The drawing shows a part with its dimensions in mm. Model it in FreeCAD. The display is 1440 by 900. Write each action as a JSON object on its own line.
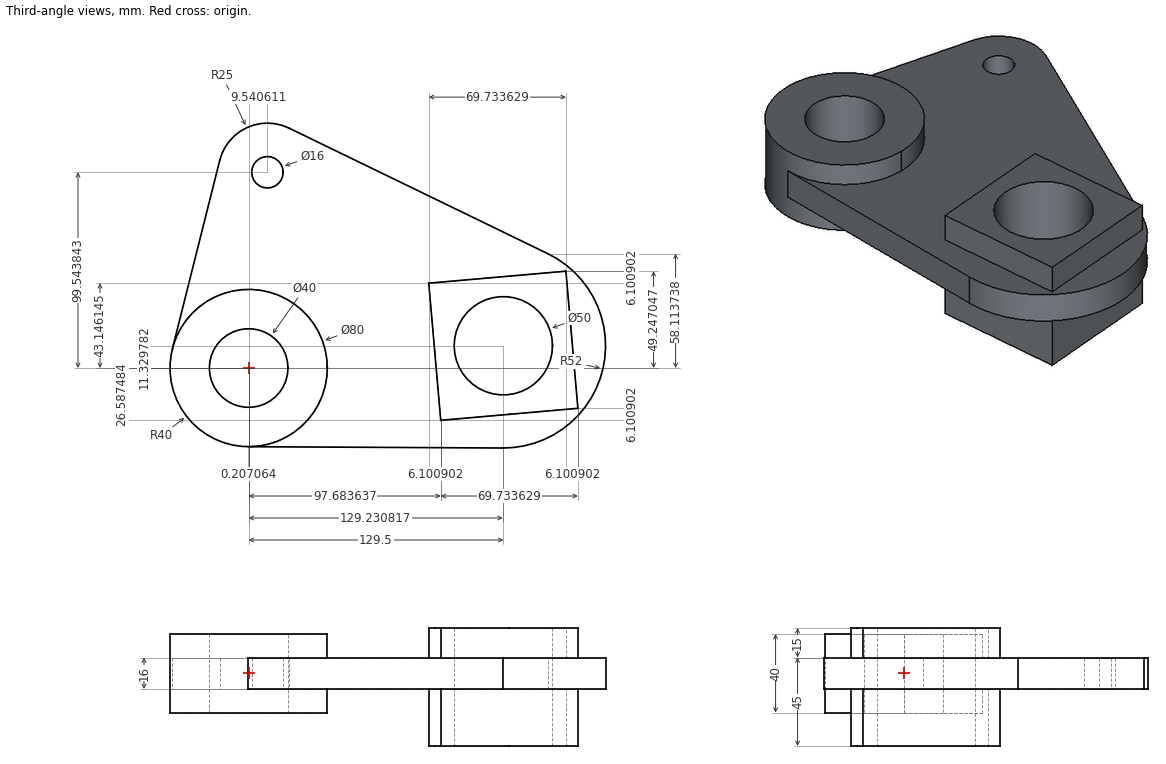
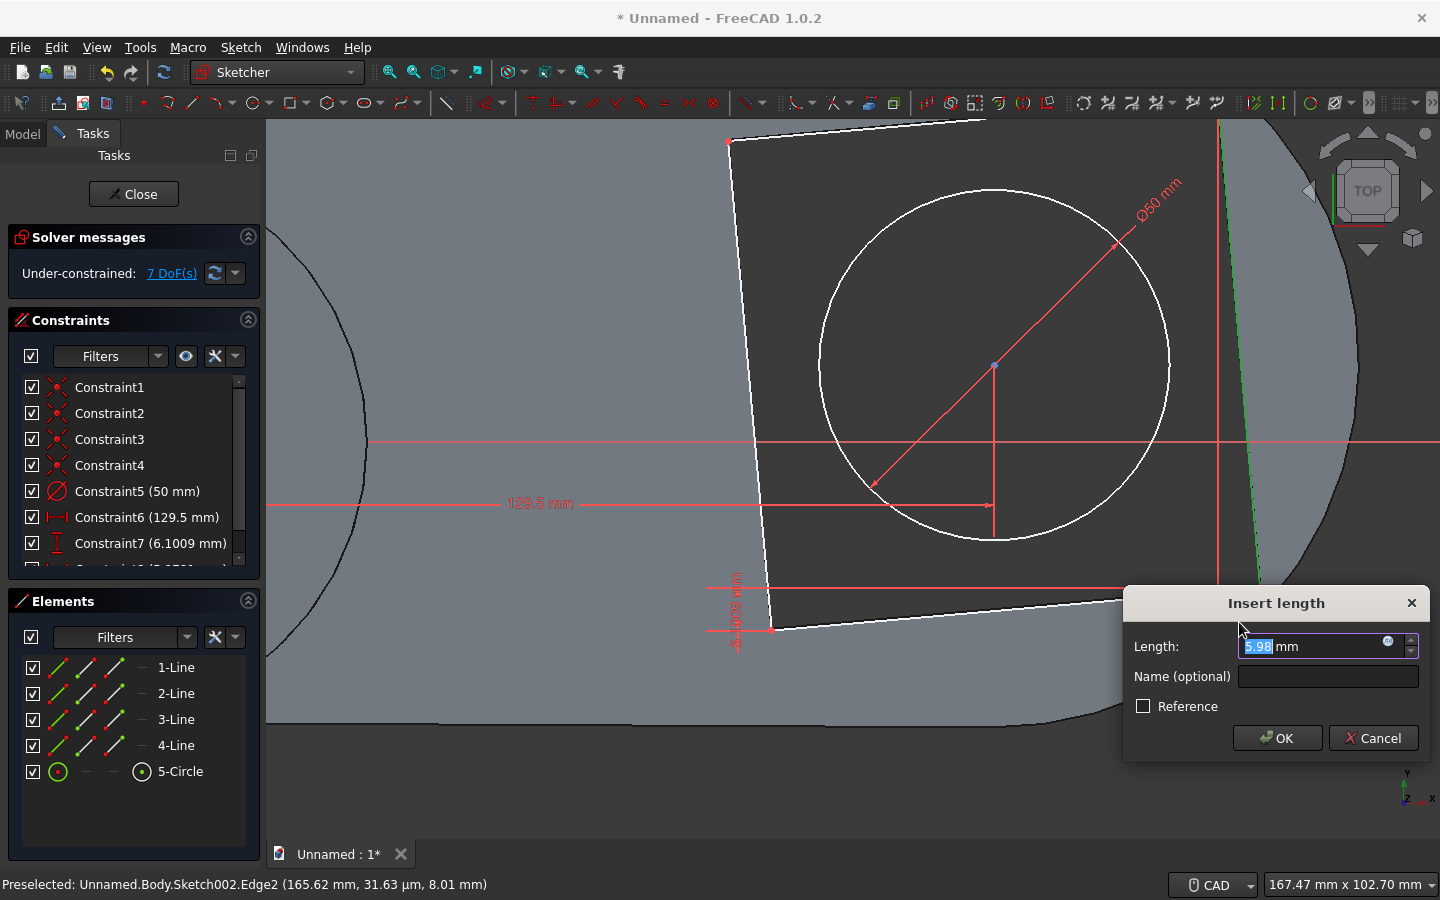
{"action": "type", "text": "6.100902"}
{"action": "key", "text": "Return"}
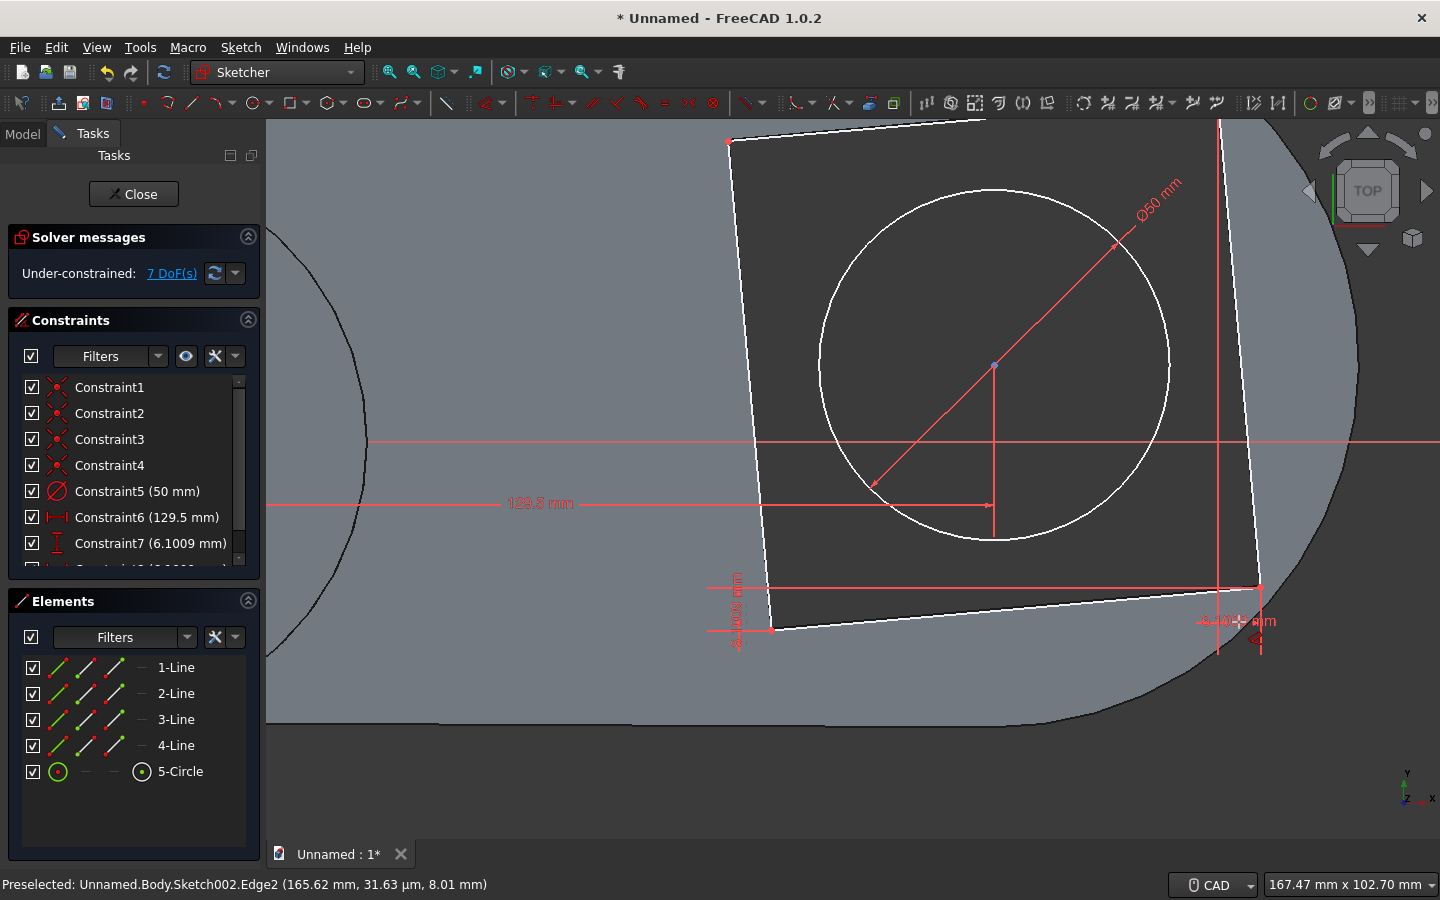
{"action": "scroll", "coordinate": [920, 620], "scroll_direction": "down", "scroll_amount": 3}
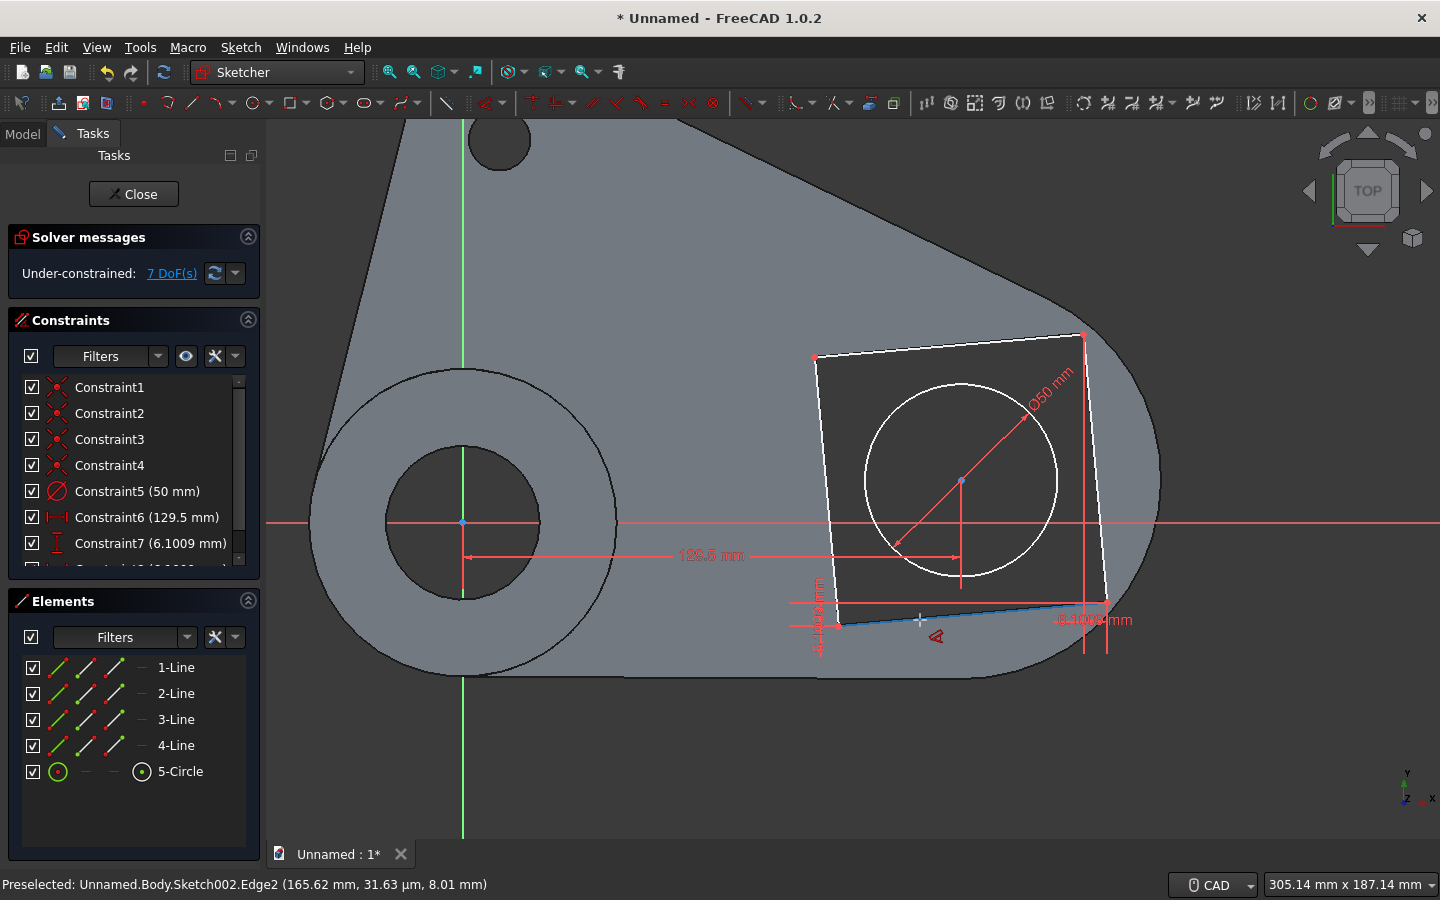
{"action": "scroll", "coordinate": [1003, 341], "scroll_direction": "up", "scroll_amount": 3}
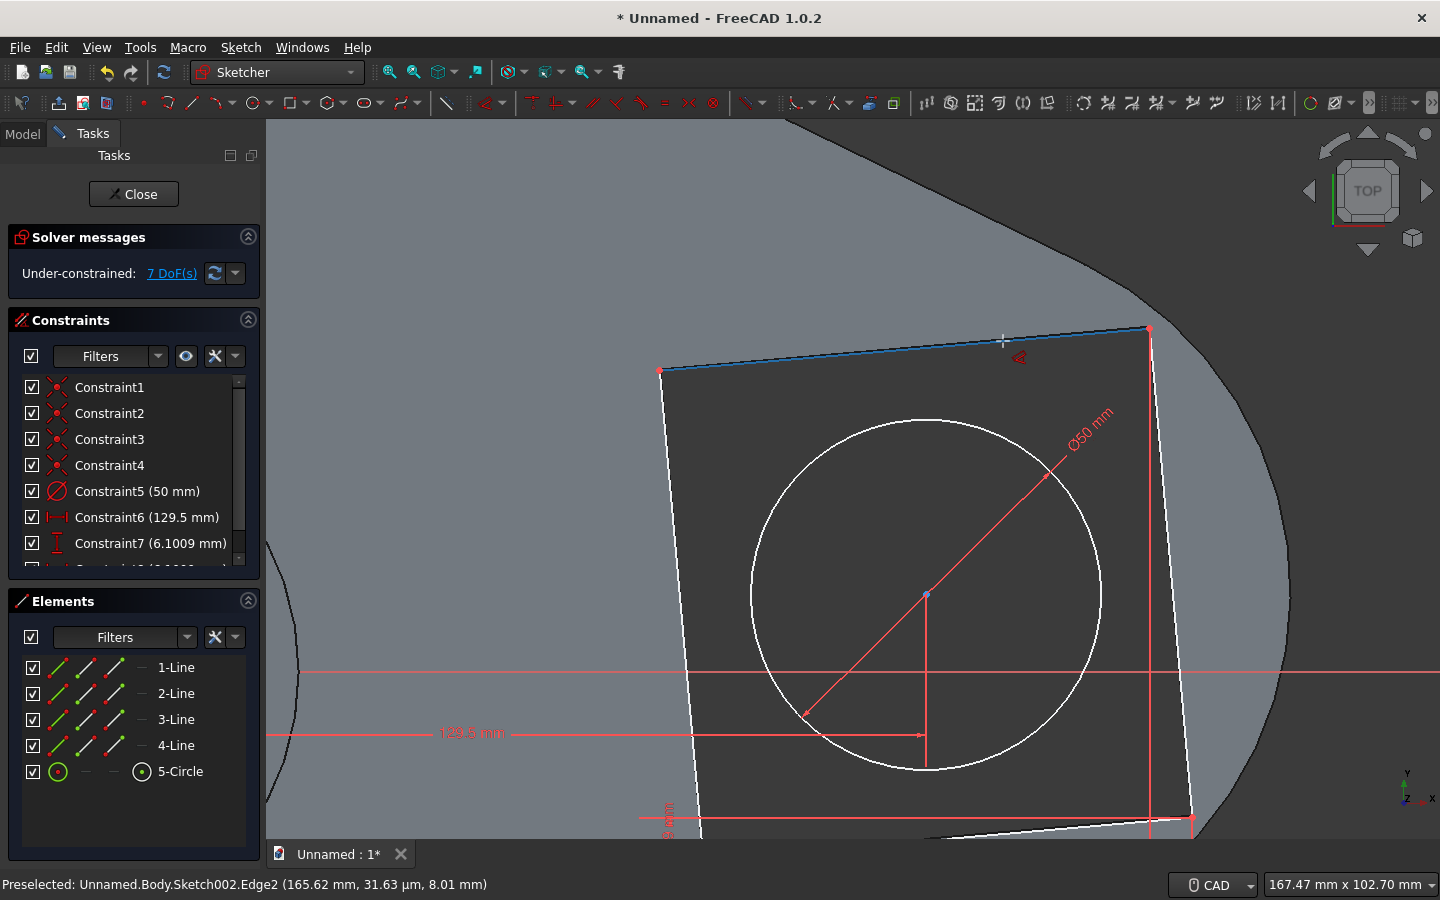
{"action": "left_click", "coordinate": [1003, 341]}
{"action": "left_click", "coordinate": [1184, 350]}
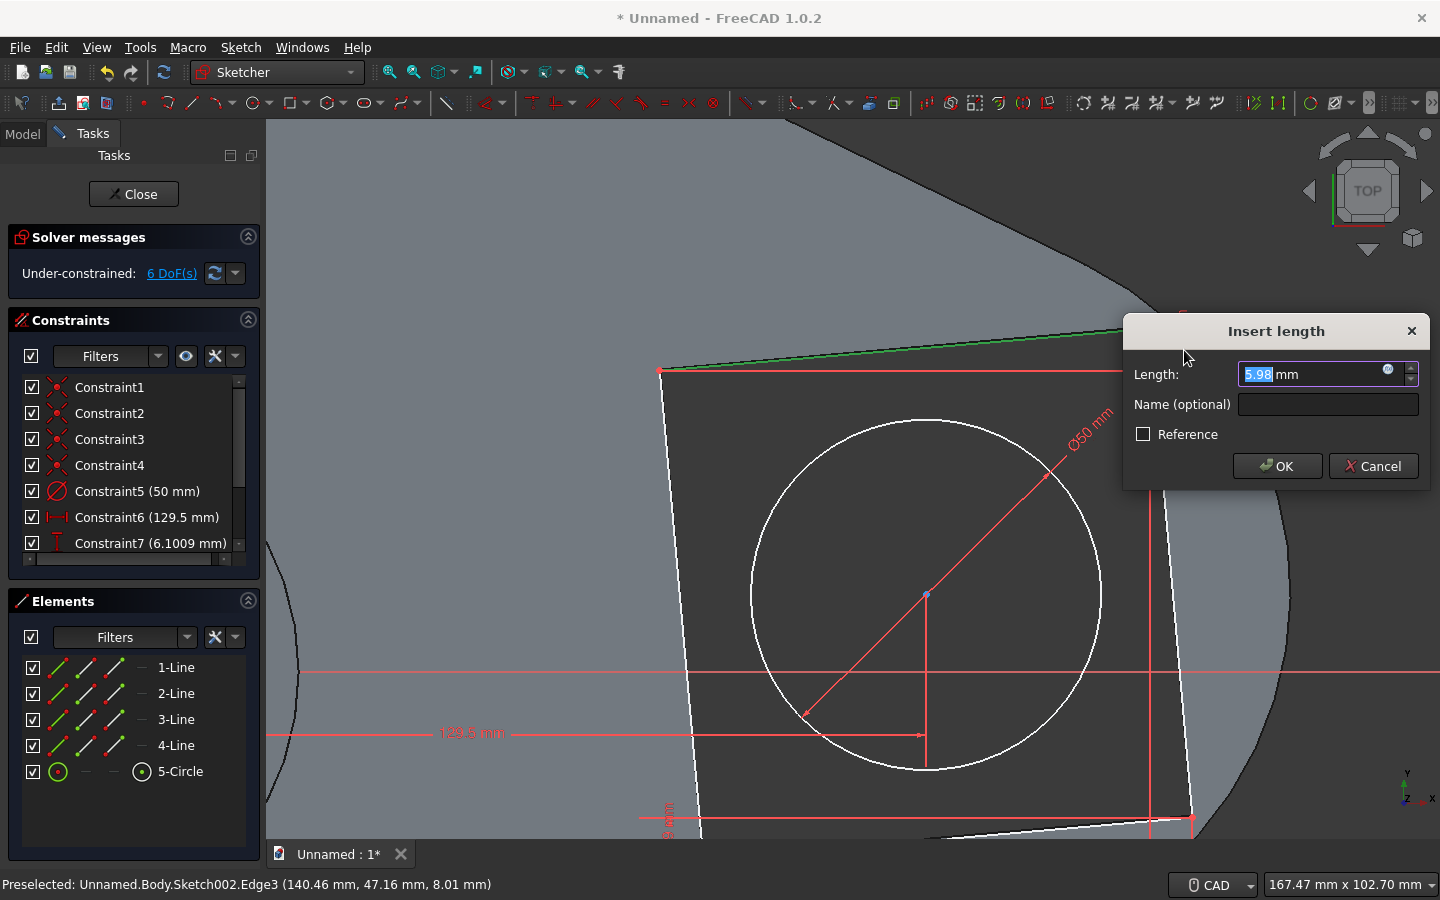
{"action": "type", "text": "6.100902"}
{"action": "key", "text": "Return"}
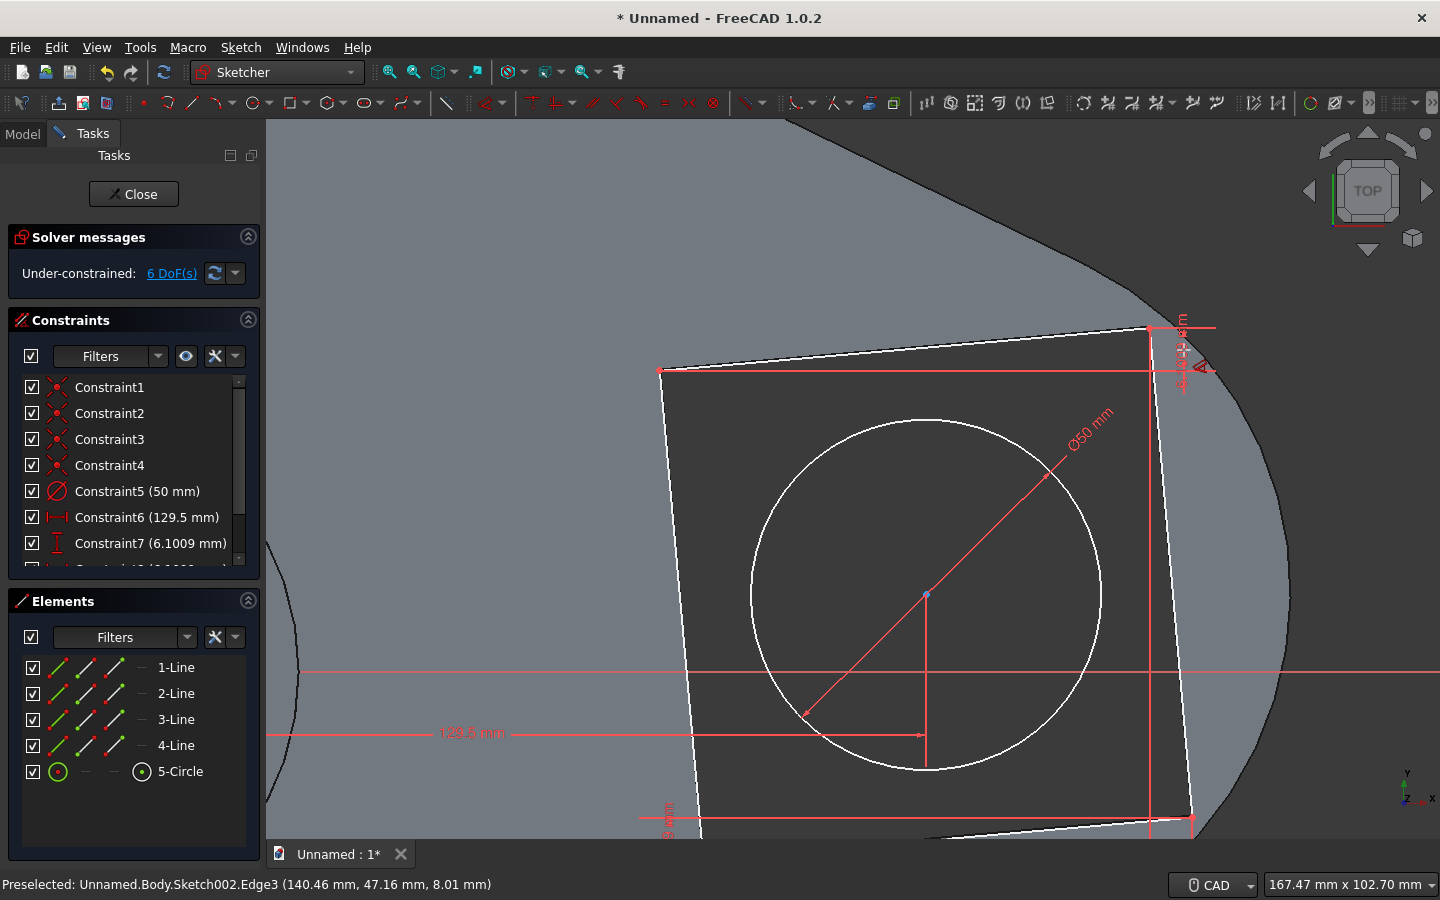
{"action": "left_click", "coordinate": [673, 518]}
{"action": "left_click", "coordinate": [682, 337]}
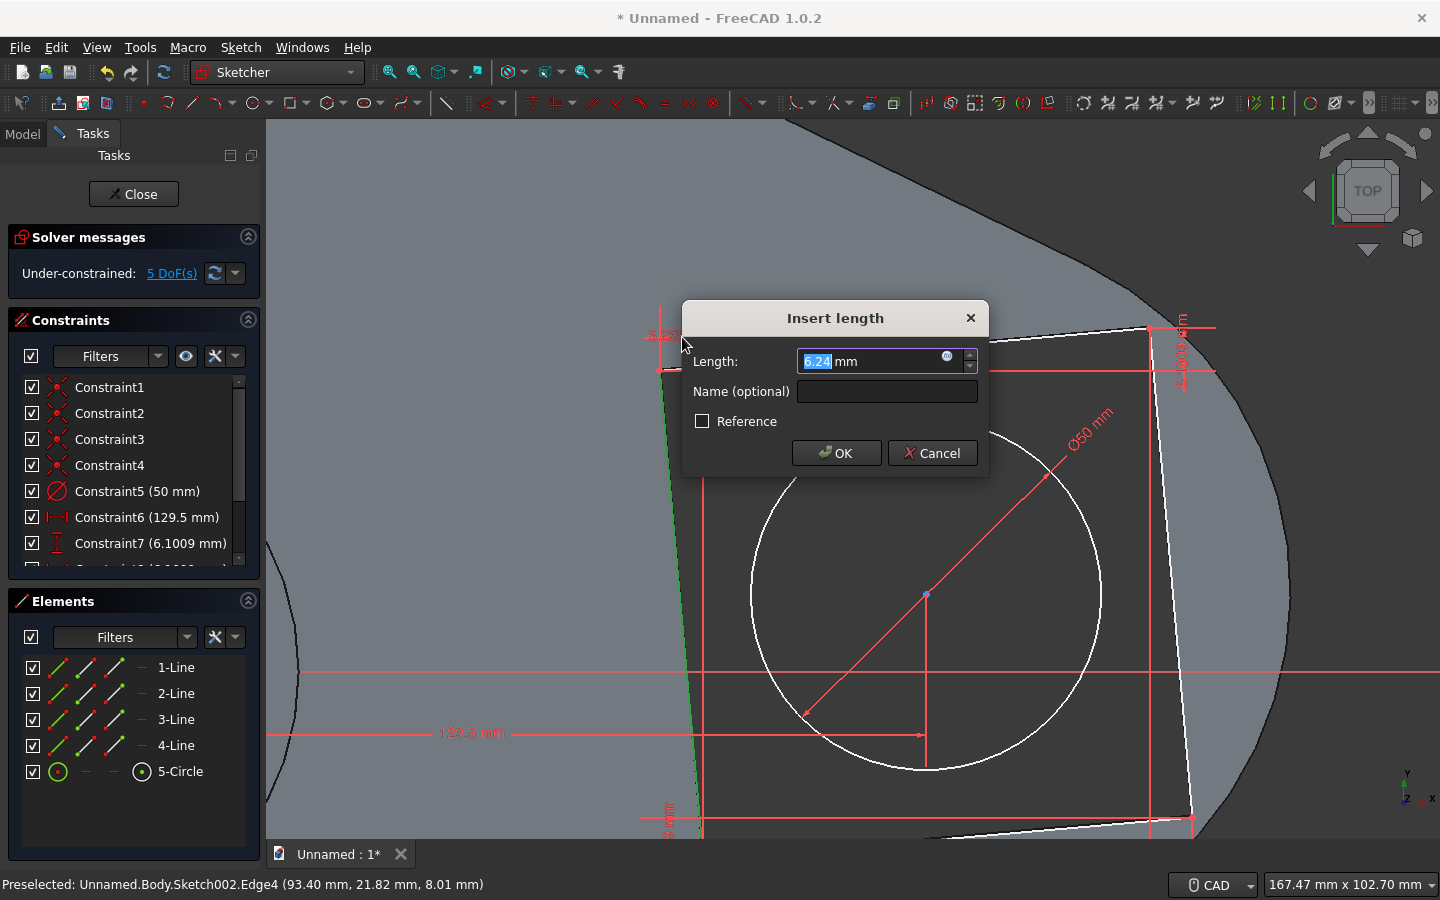
{"action": "type", "text": "6.100902"}
{"action": "key", "text": "Return"}